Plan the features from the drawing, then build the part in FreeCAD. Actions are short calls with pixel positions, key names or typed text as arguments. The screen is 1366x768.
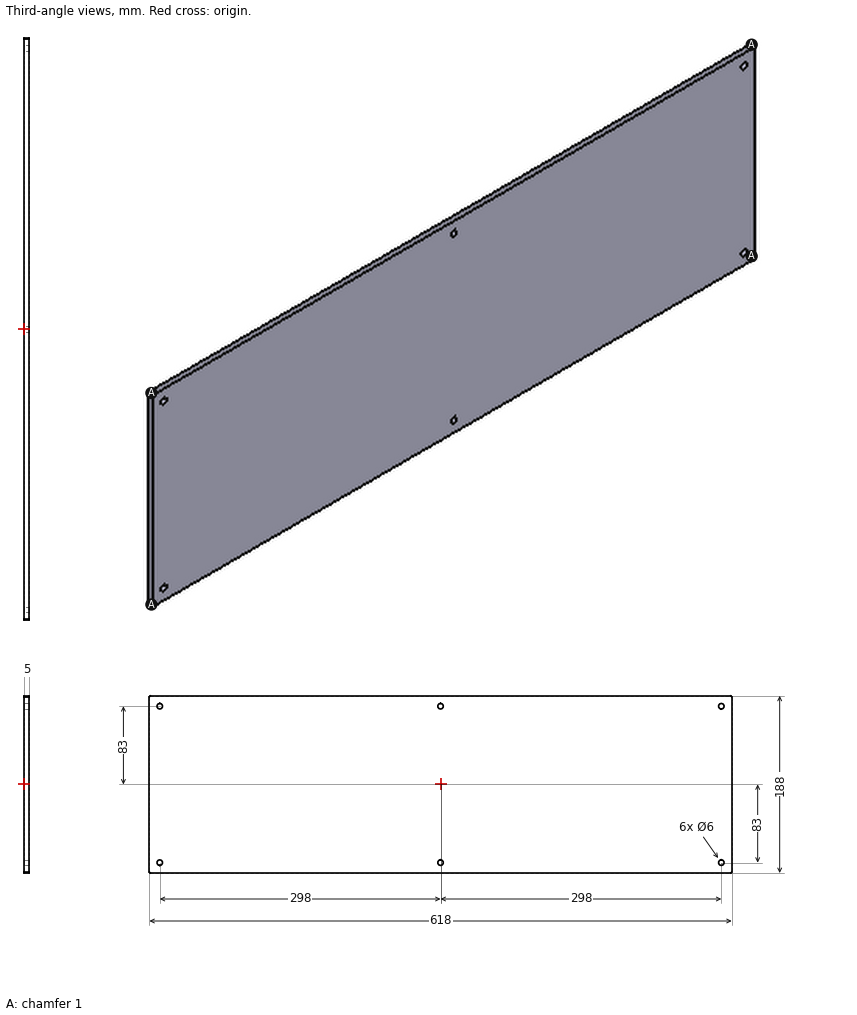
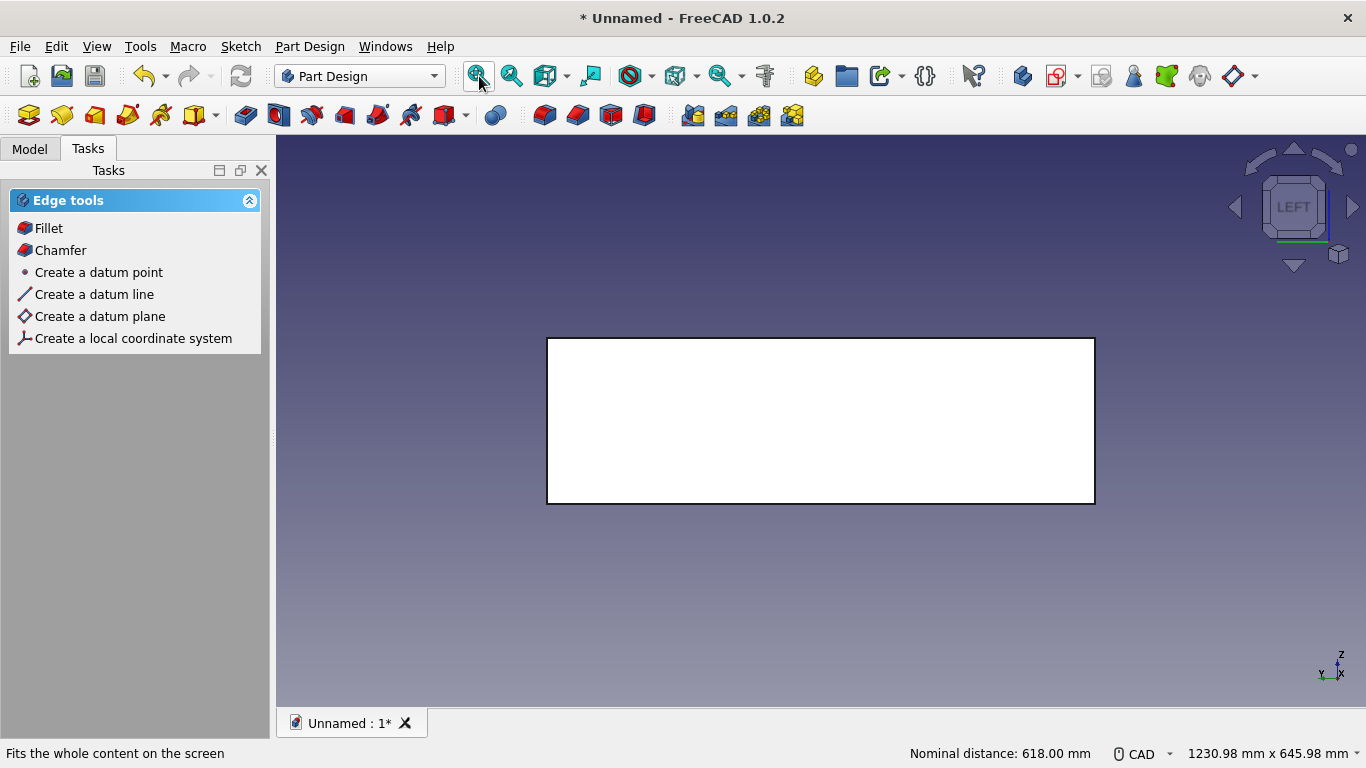
key(v)
key(3)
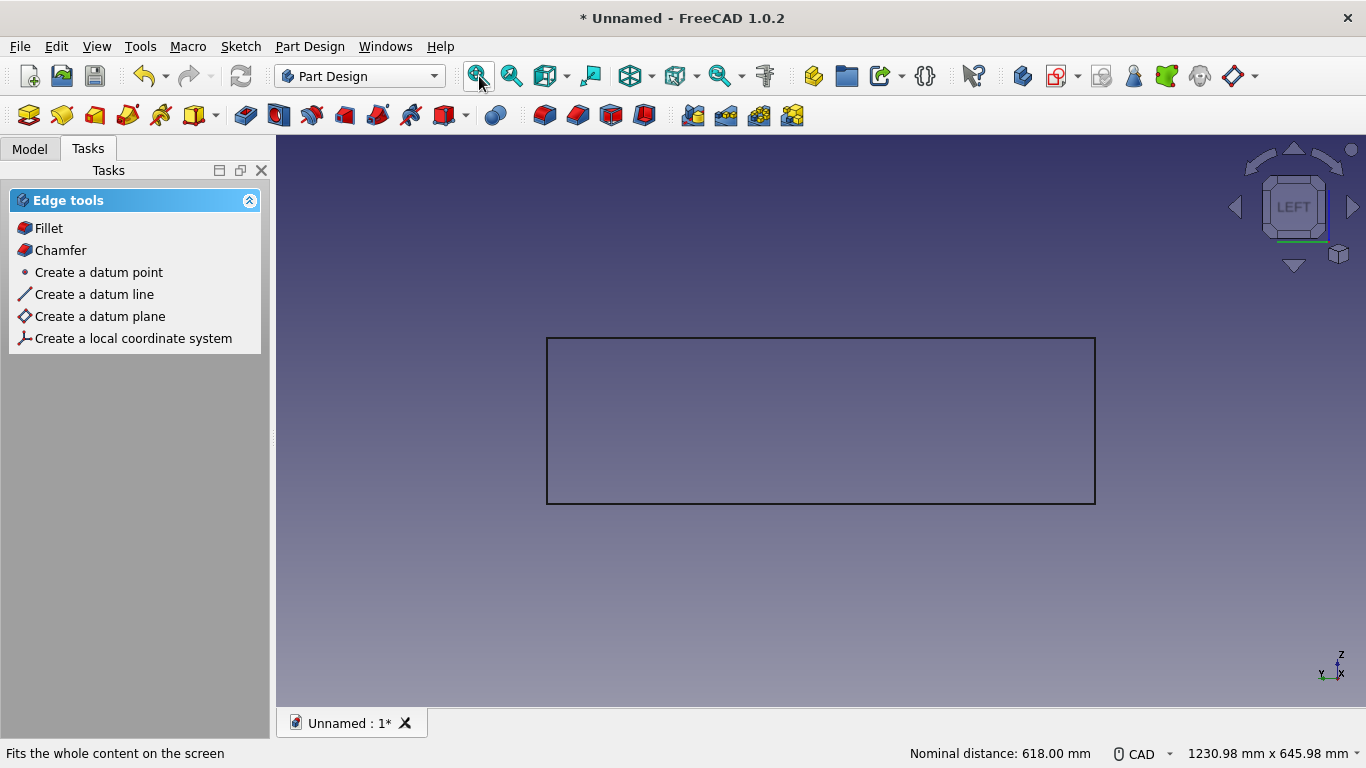
key(0)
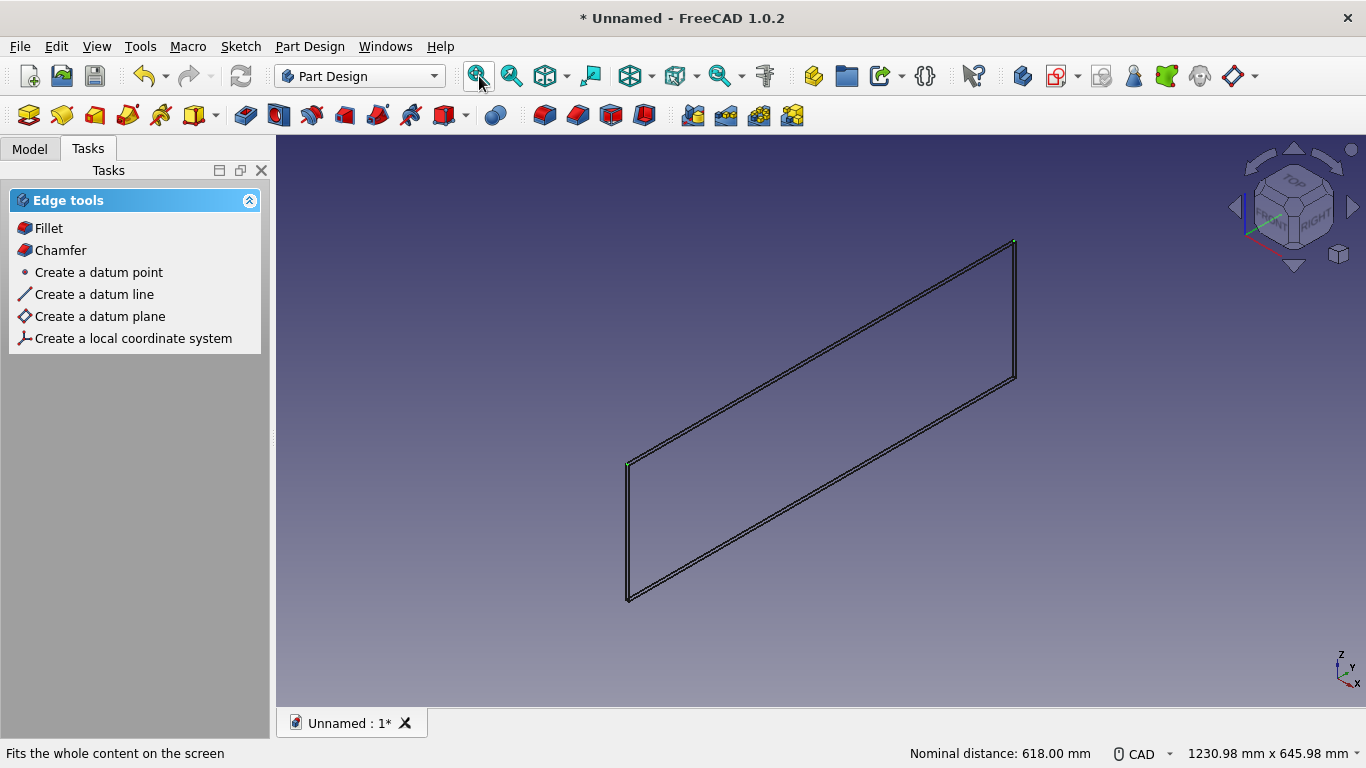
scroll(1014, 376, up, 12)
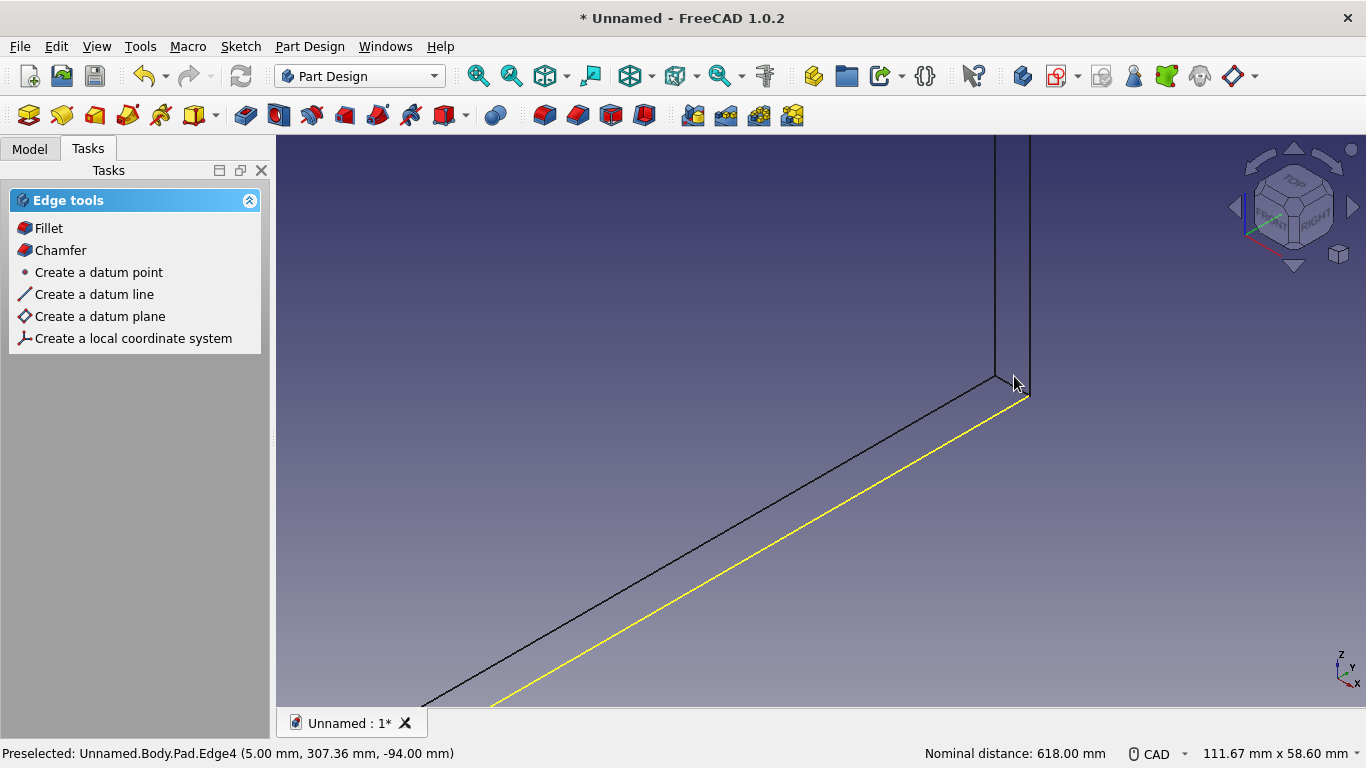
click(1012, 385, ctrl)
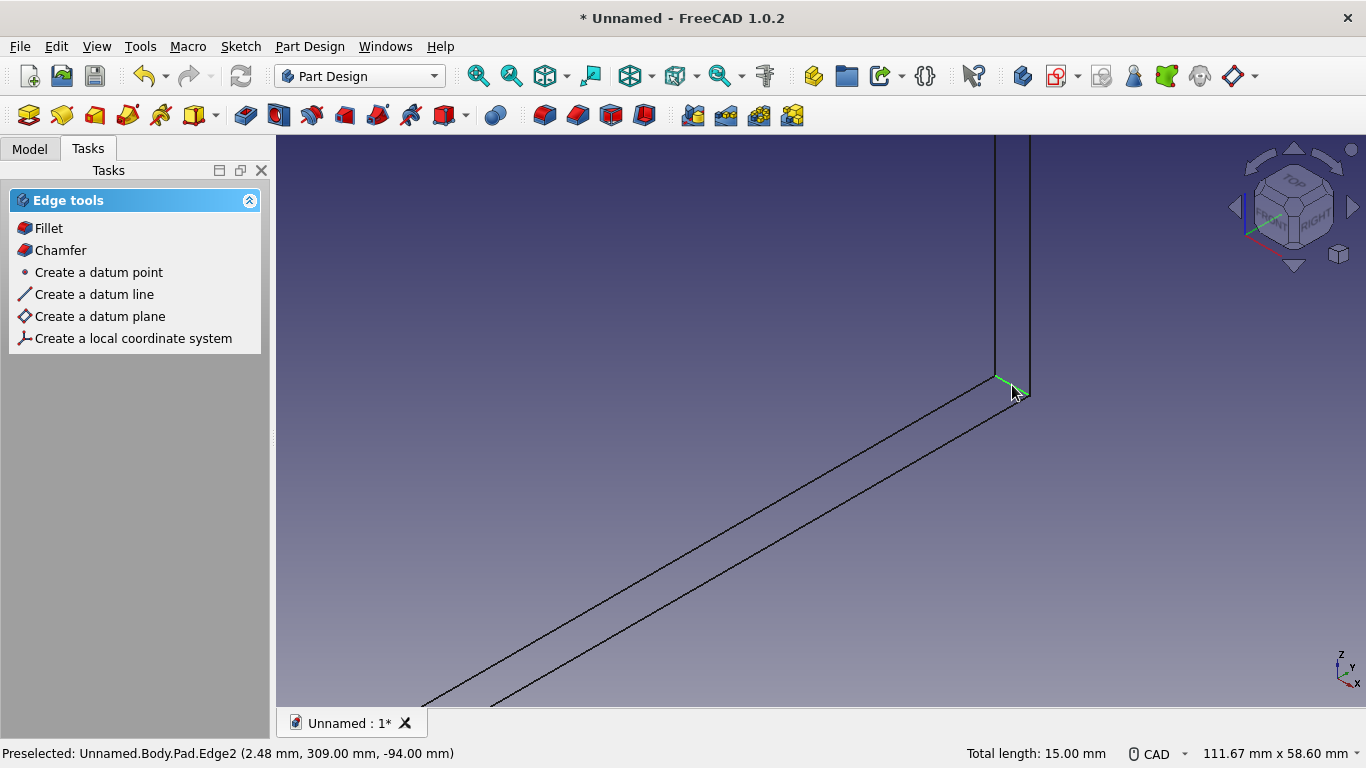
click(479, 76)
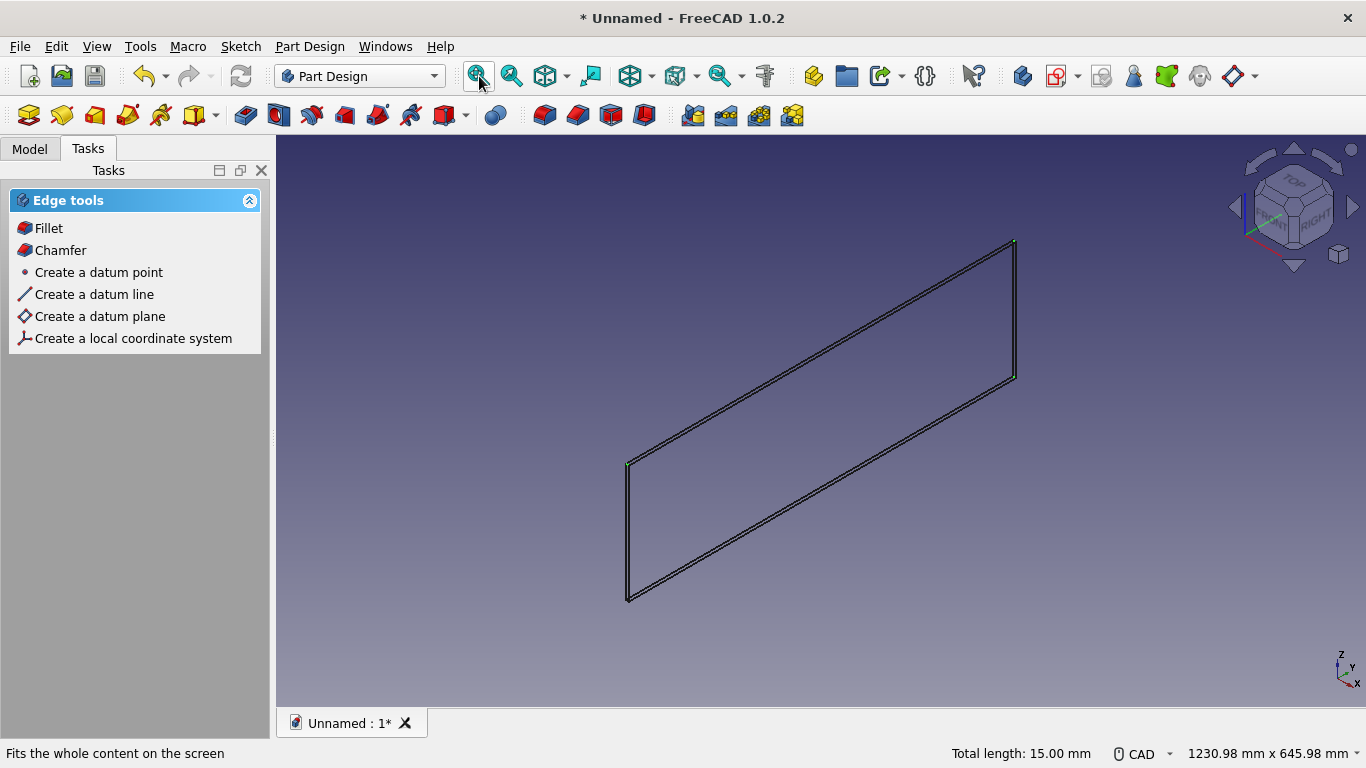
key(2)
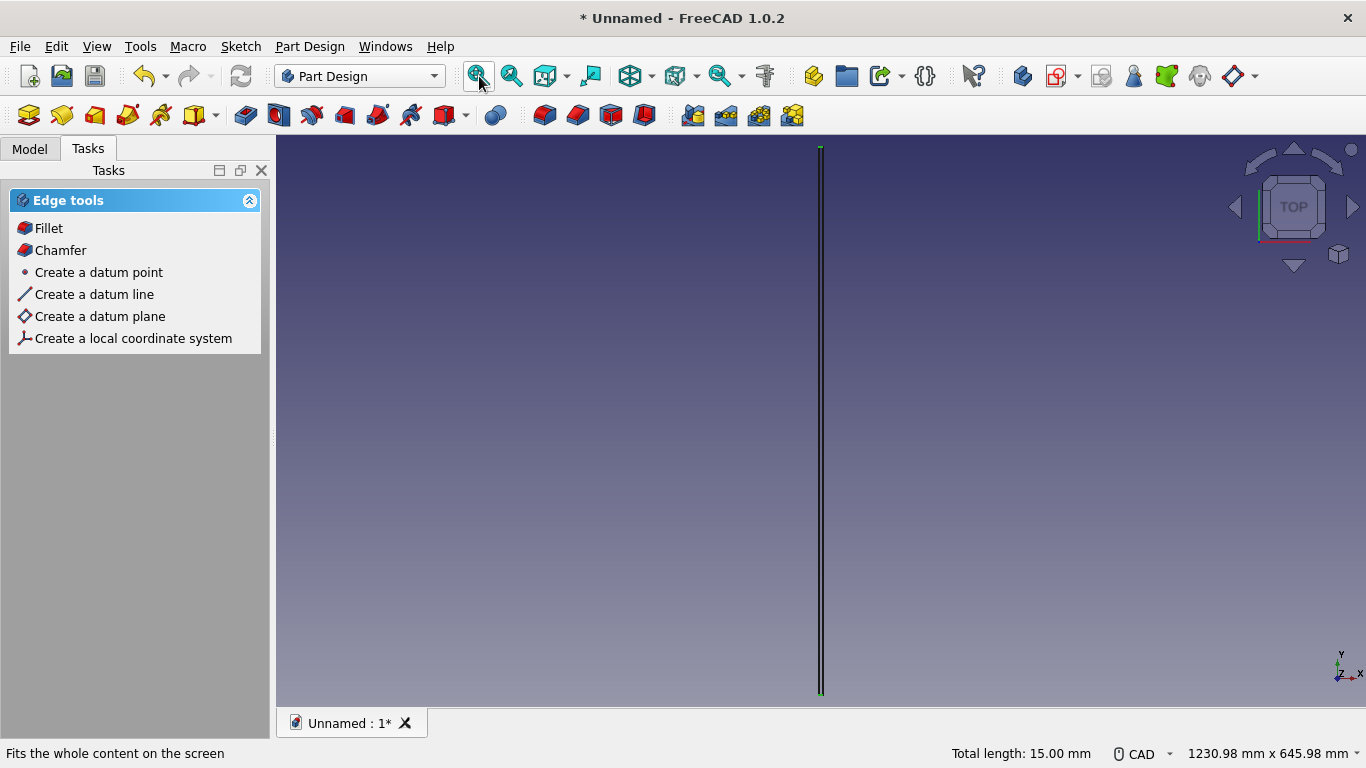
key(1)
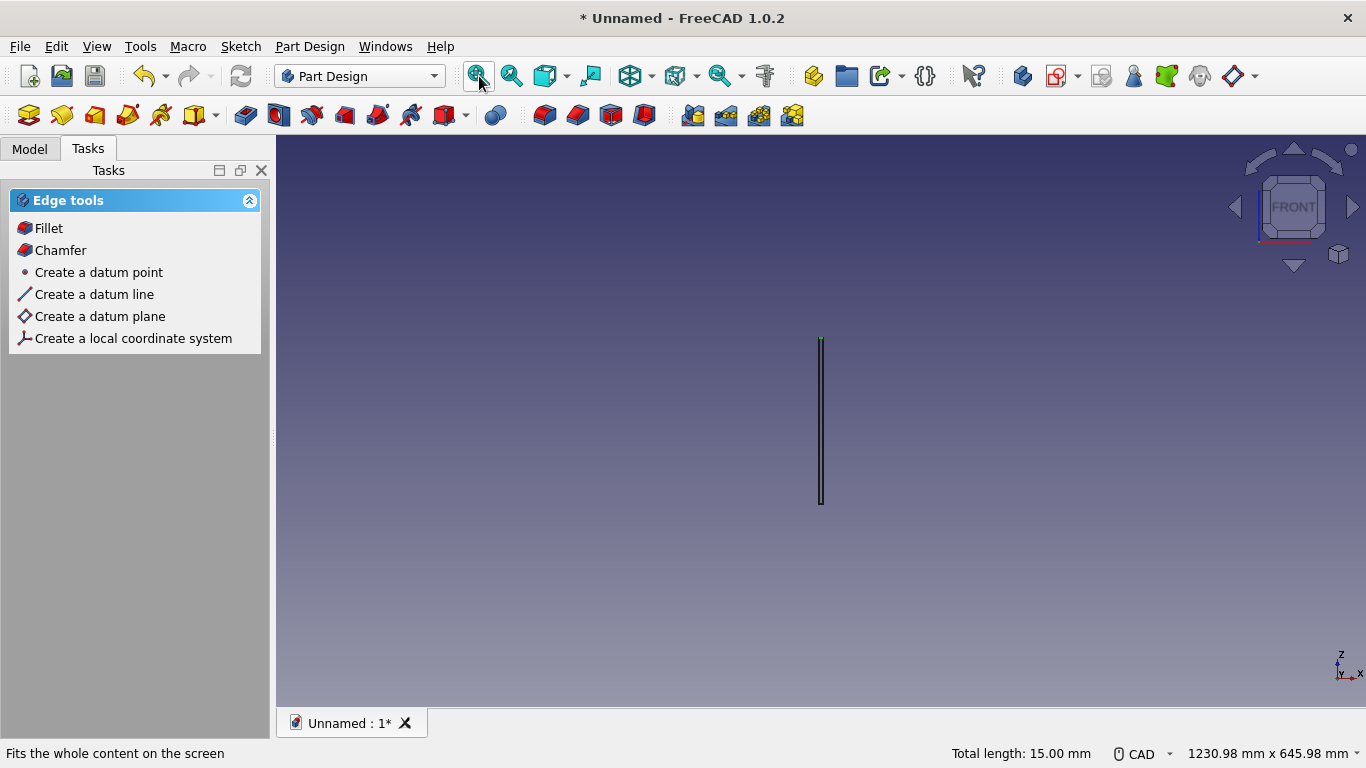
click(479, 76)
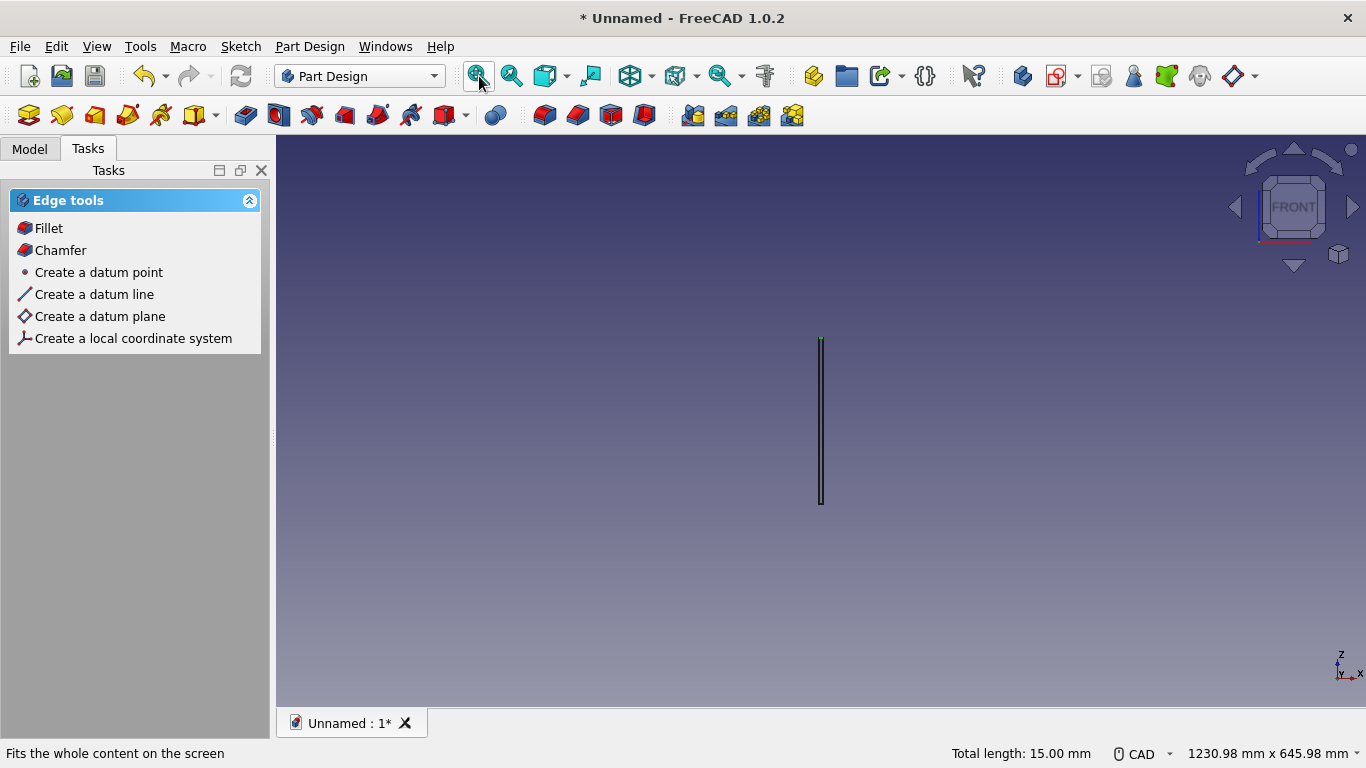
click(821, 503, ctrl)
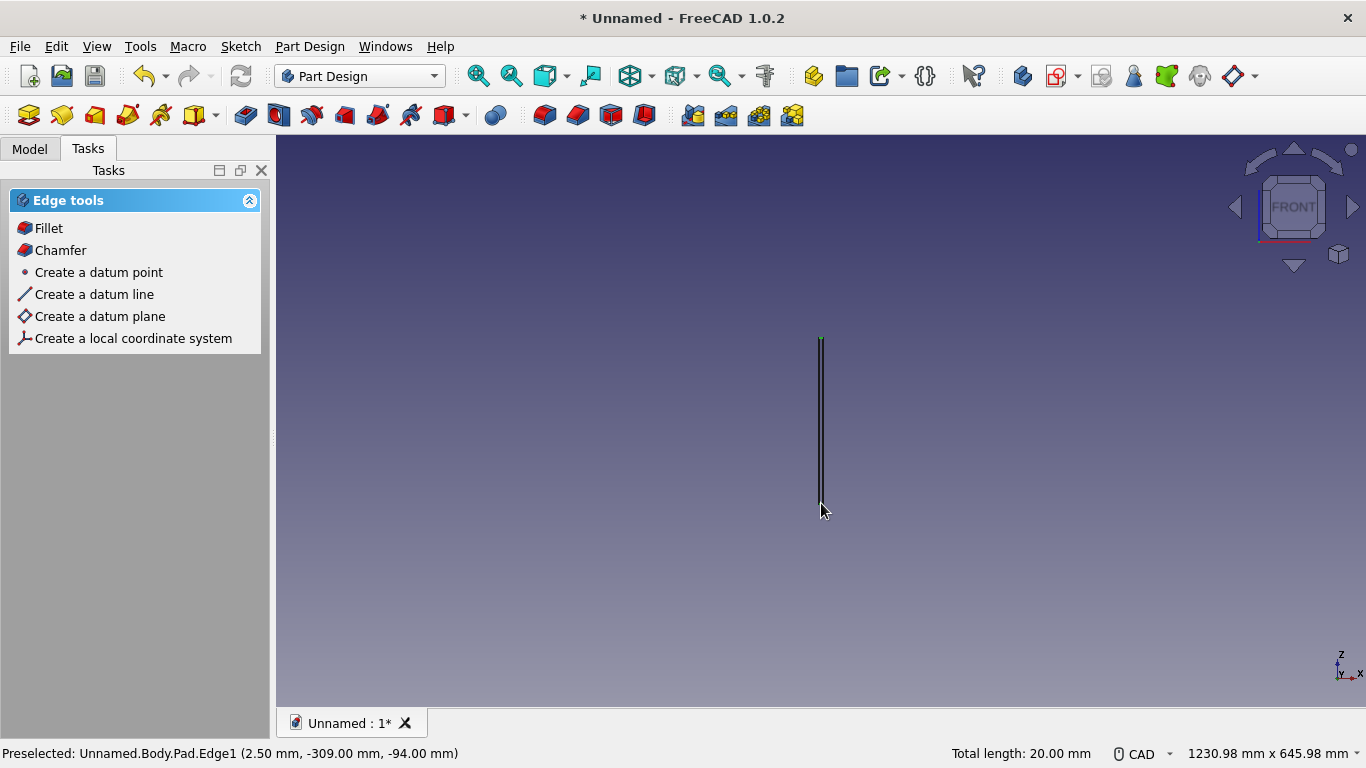
key(v)
key(1)